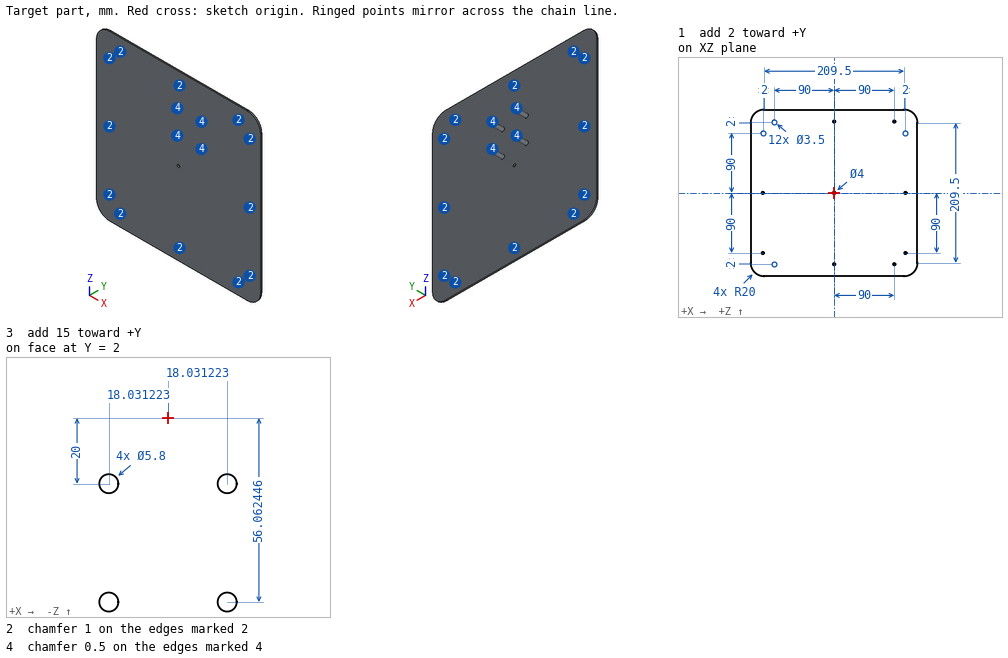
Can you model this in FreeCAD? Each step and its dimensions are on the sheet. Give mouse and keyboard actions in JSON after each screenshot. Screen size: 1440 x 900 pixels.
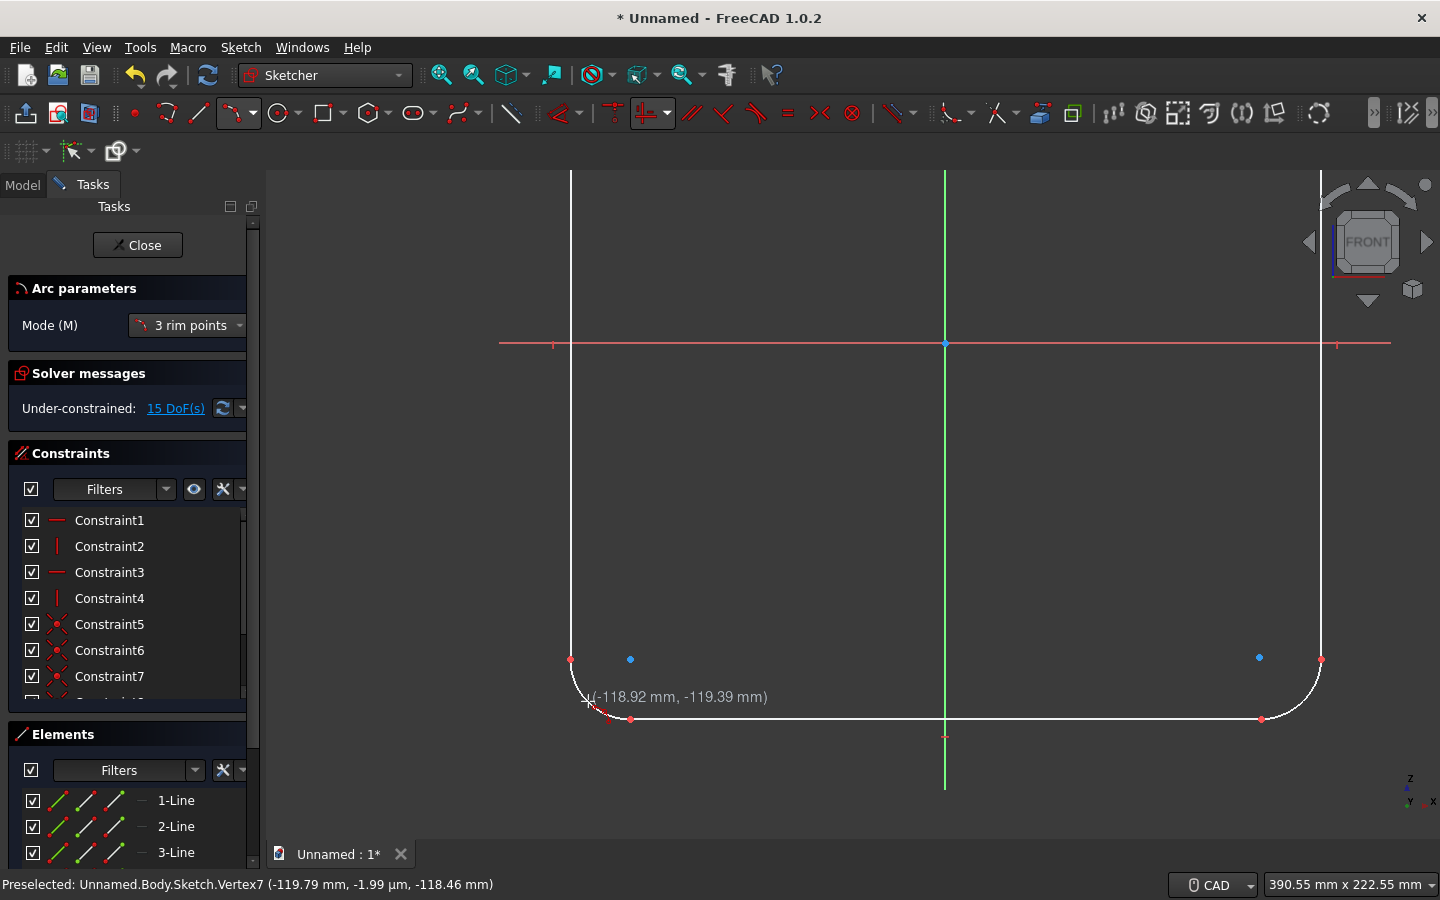
{"action": "scroll", "coordinate": [589, 701], "scroll_direction": "down", "scroll_amount": 3}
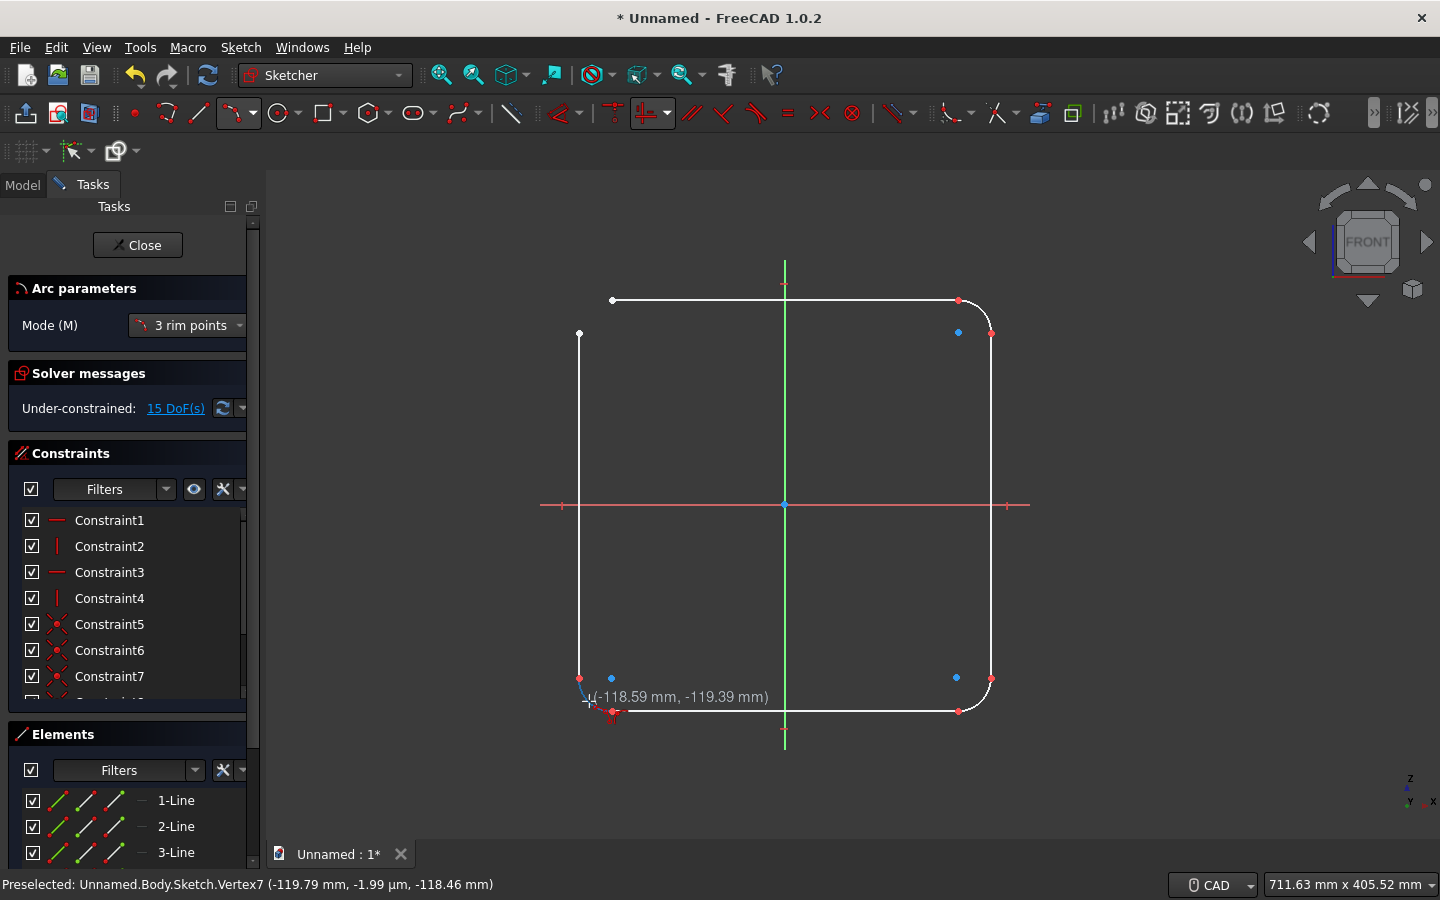
{"action": "left_click", "coordinate": [579, 333]}
{"action": "left_click", "coordinate": [612, 300]}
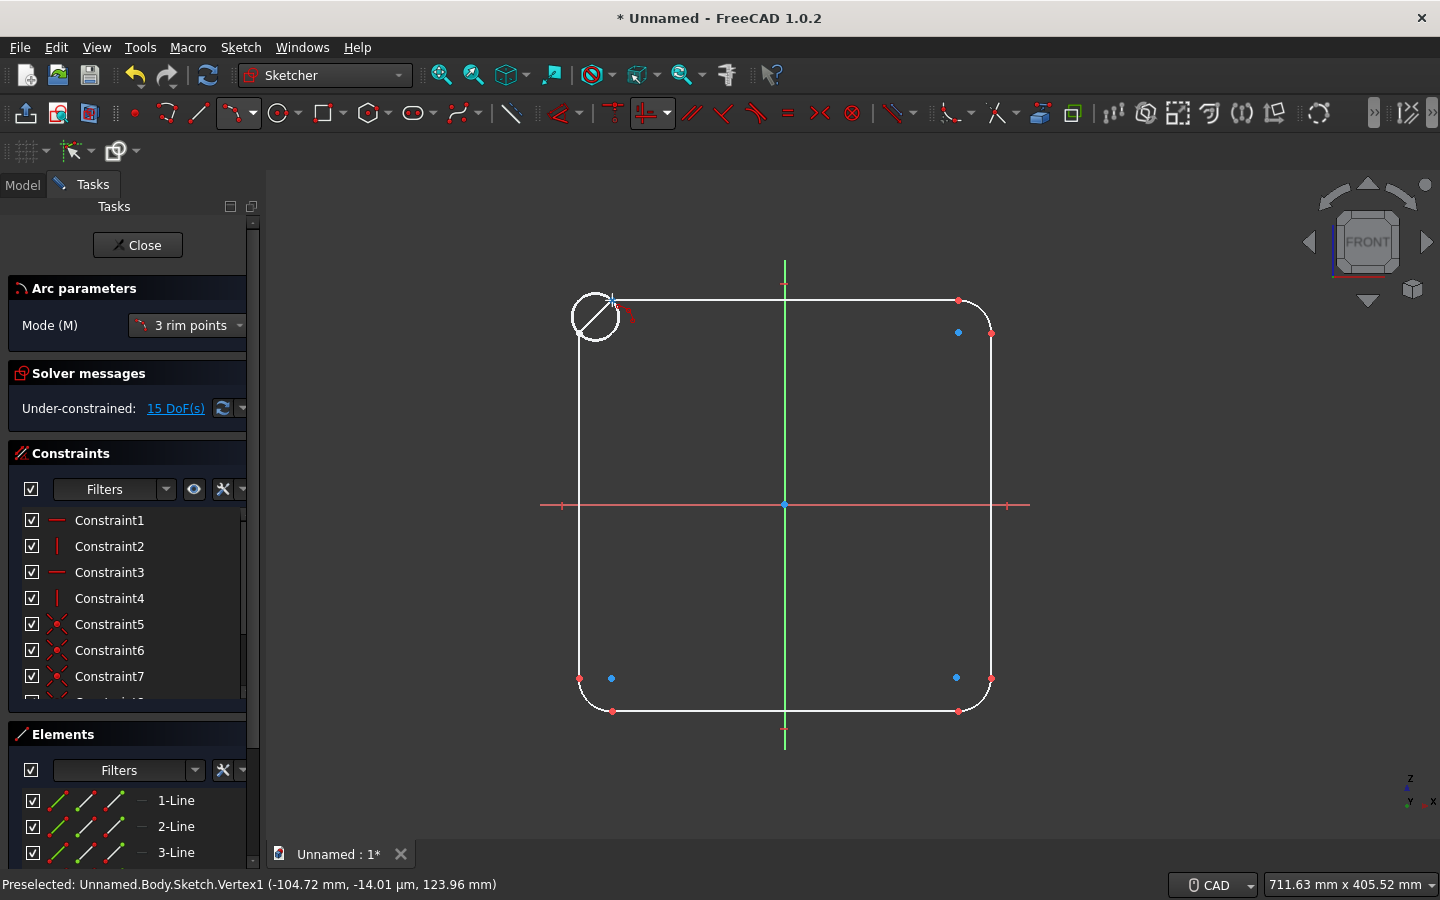
{"action": "scroll", "coordinate": [589, 309], "scroll_direction": "up", "scroll_amount": 3}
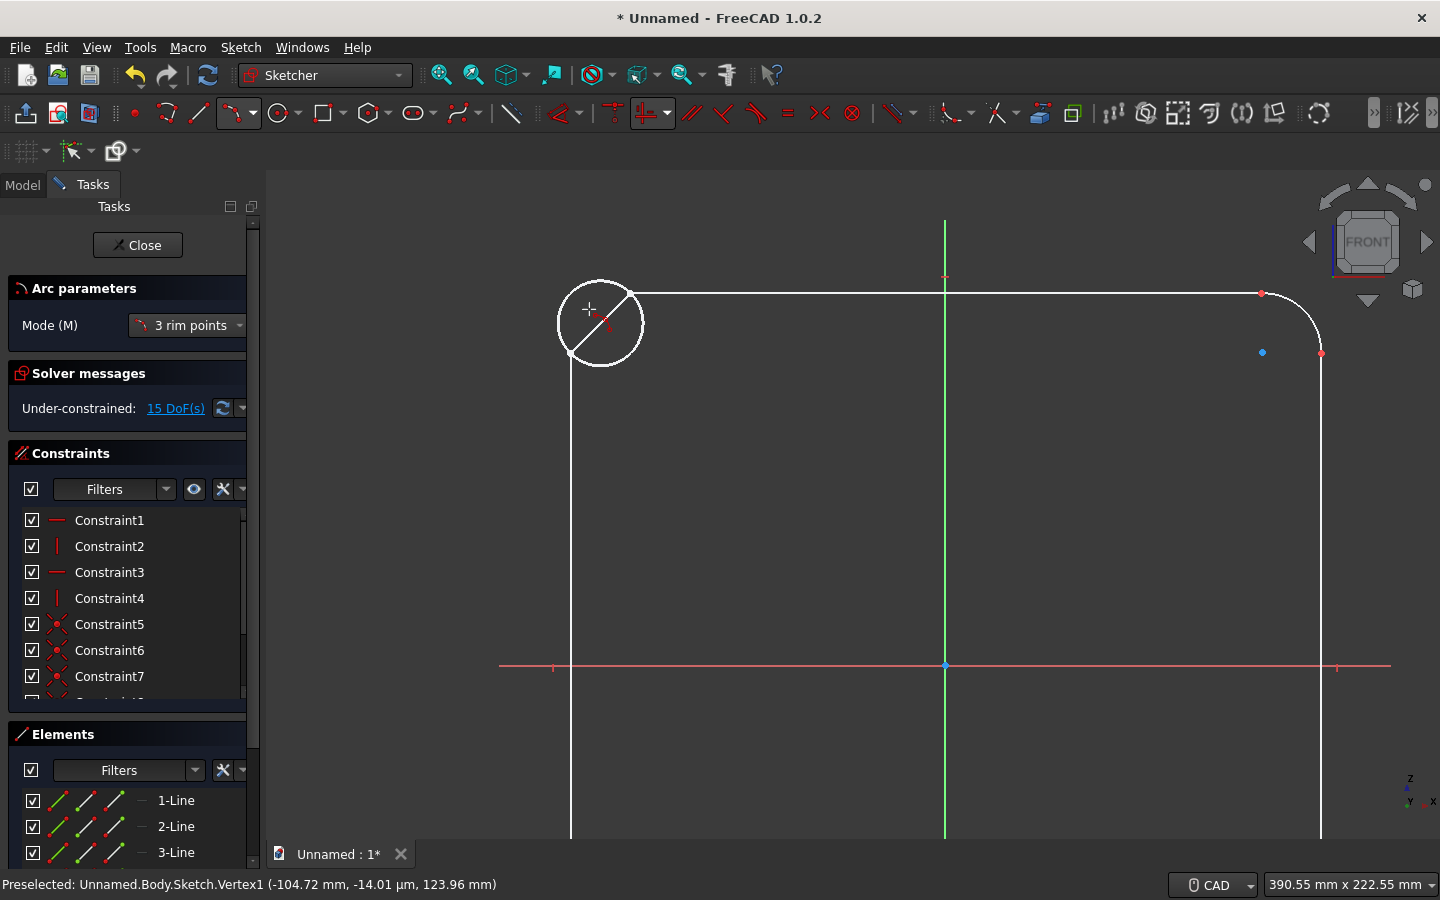
{"action": "left_click", "coordinate": [588, 308]}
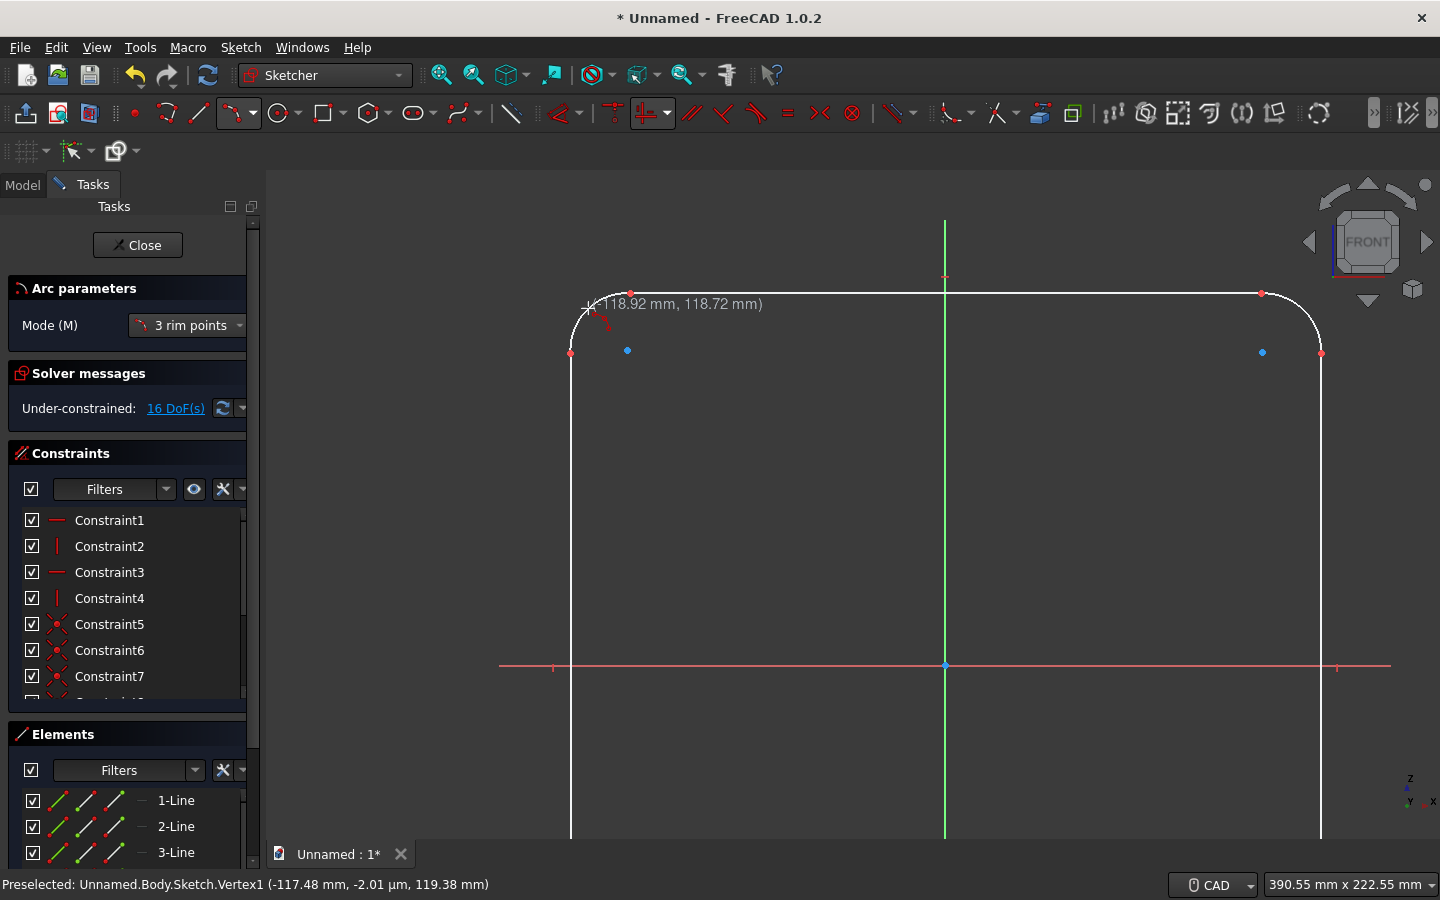
{"action": "key", "text": "g c"}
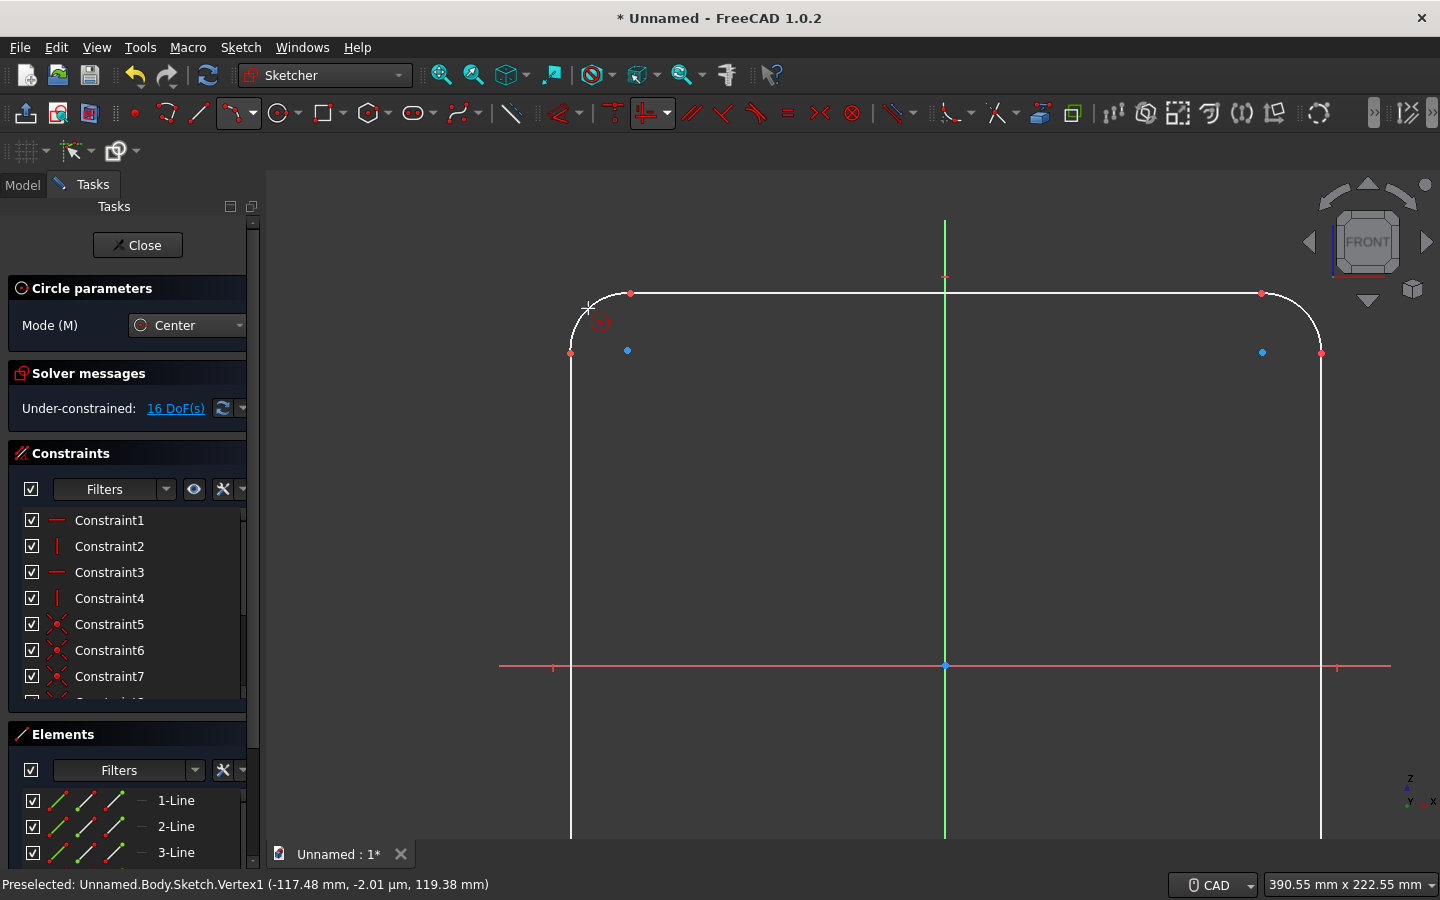
{"action": "scroll", "coordinate": [675, 345], "scroll_direction": "up", "scroll_amount": 8}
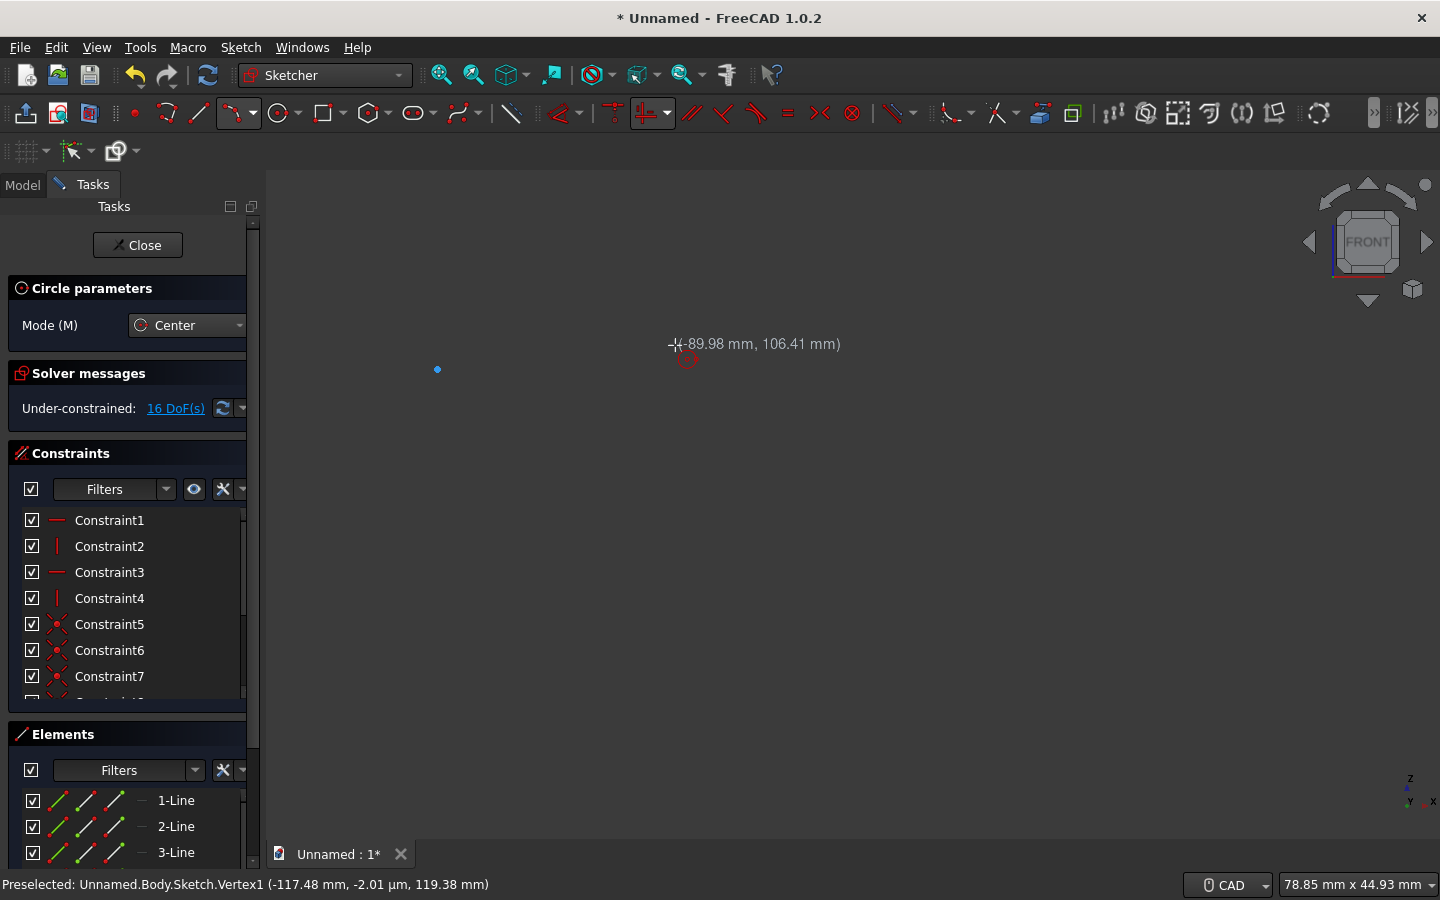
{"action": "scroll", "coordinate": [631, 326], "scroll_direction": "down", "scroll_amount": 11}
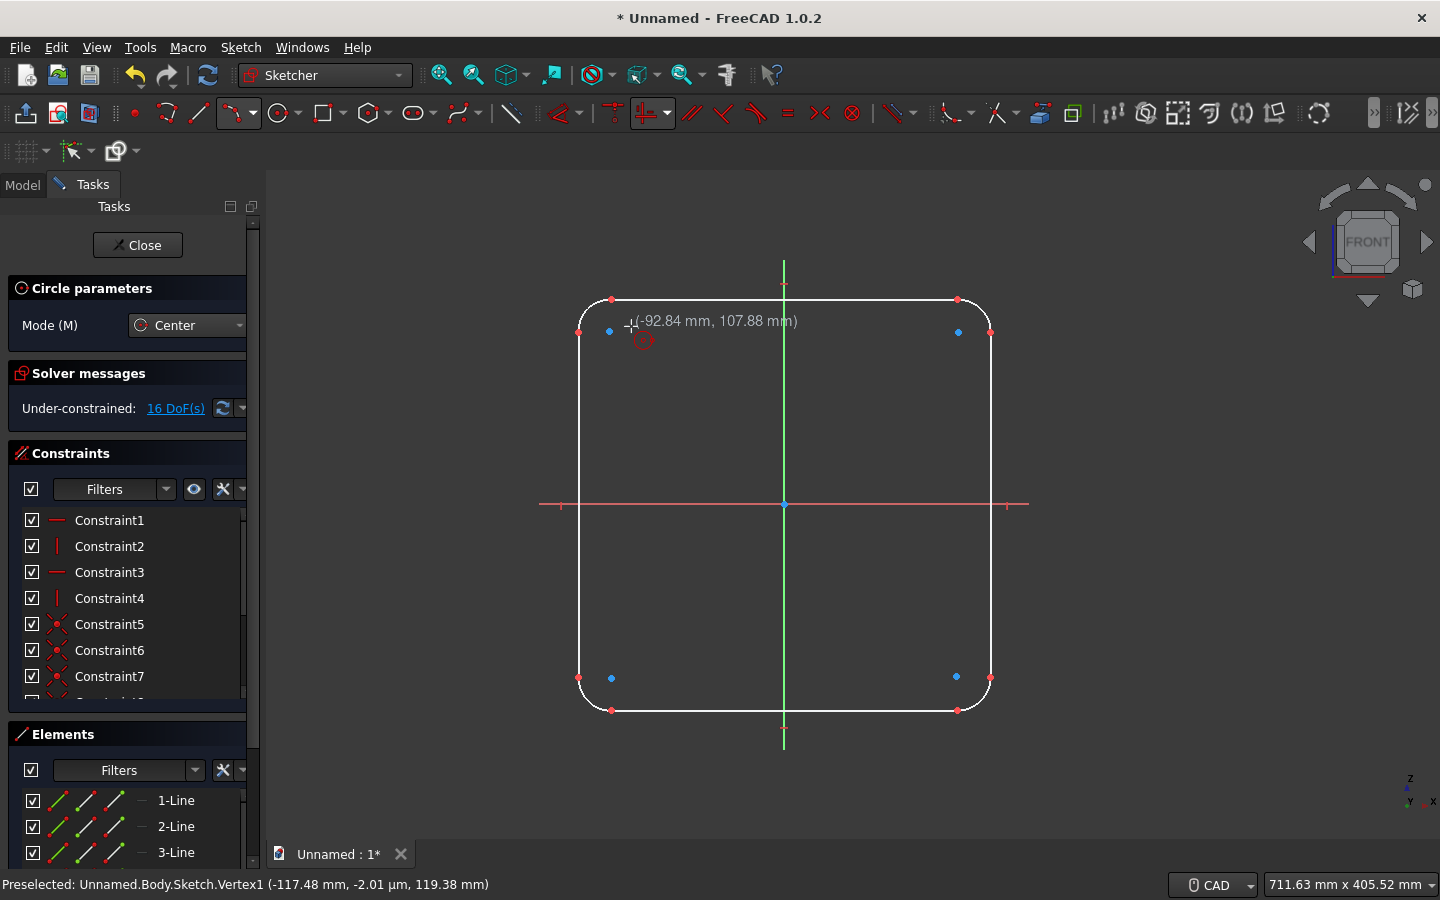
{"action": "left_click", "coordinate": [636, 328]}
{"action": "mouse_move", "coordinate": [638, 326]}